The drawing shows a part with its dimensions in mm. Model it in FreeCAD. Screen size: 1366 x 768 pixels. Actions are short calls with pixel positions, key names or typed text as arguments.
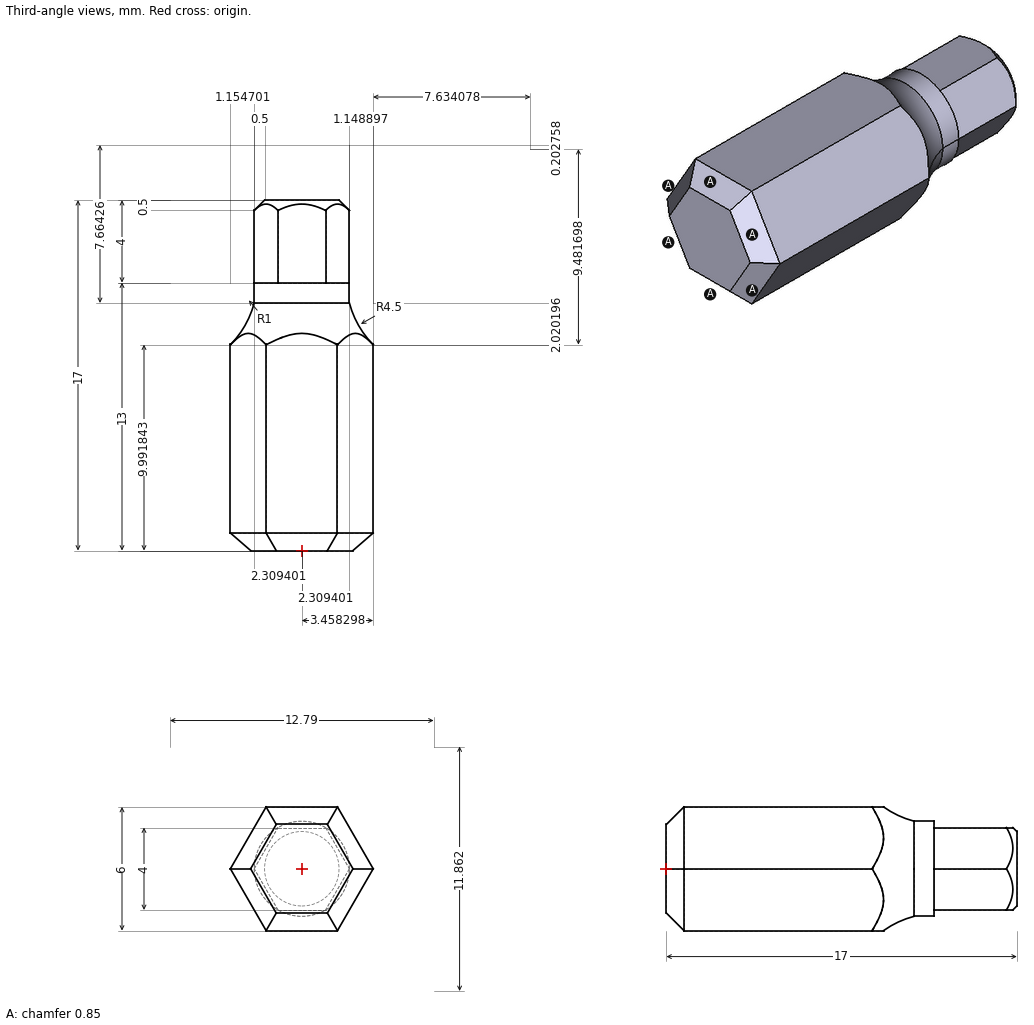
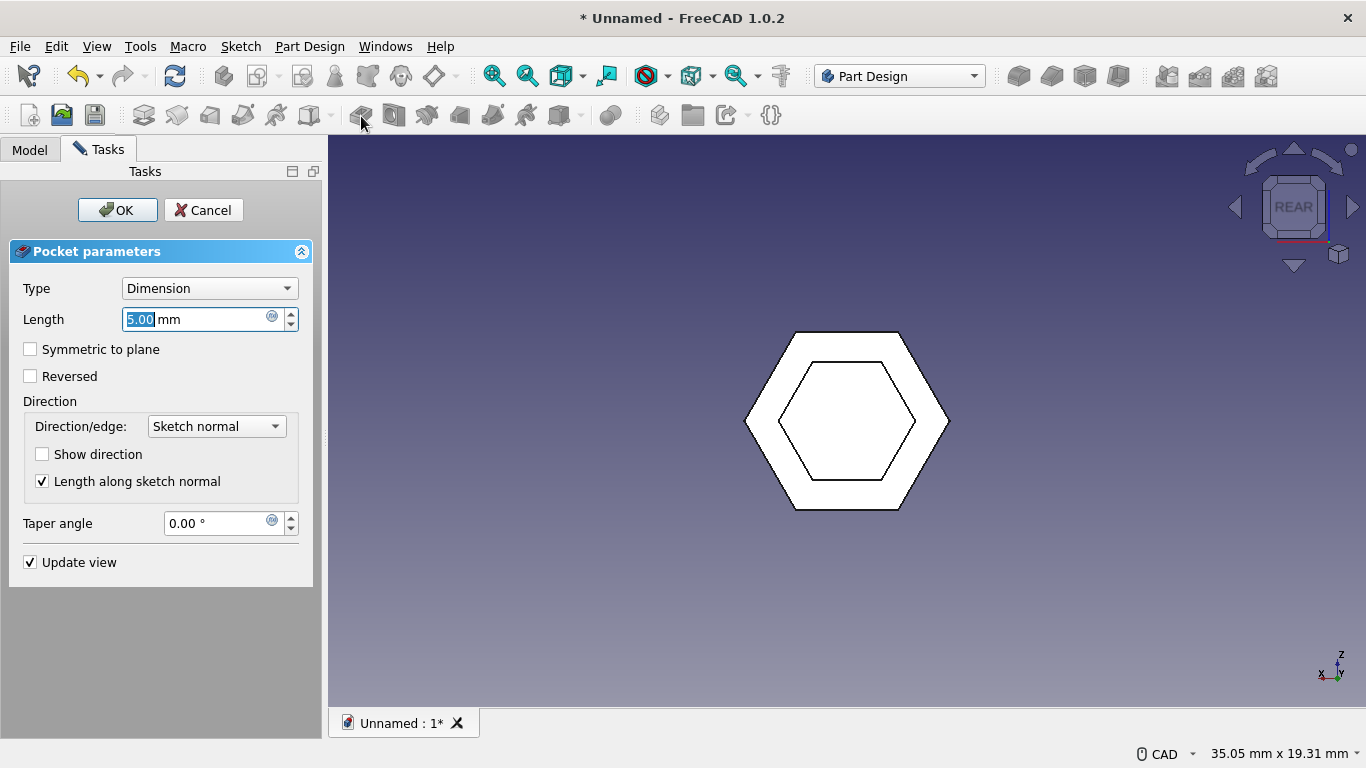
text(4)
key(Tab)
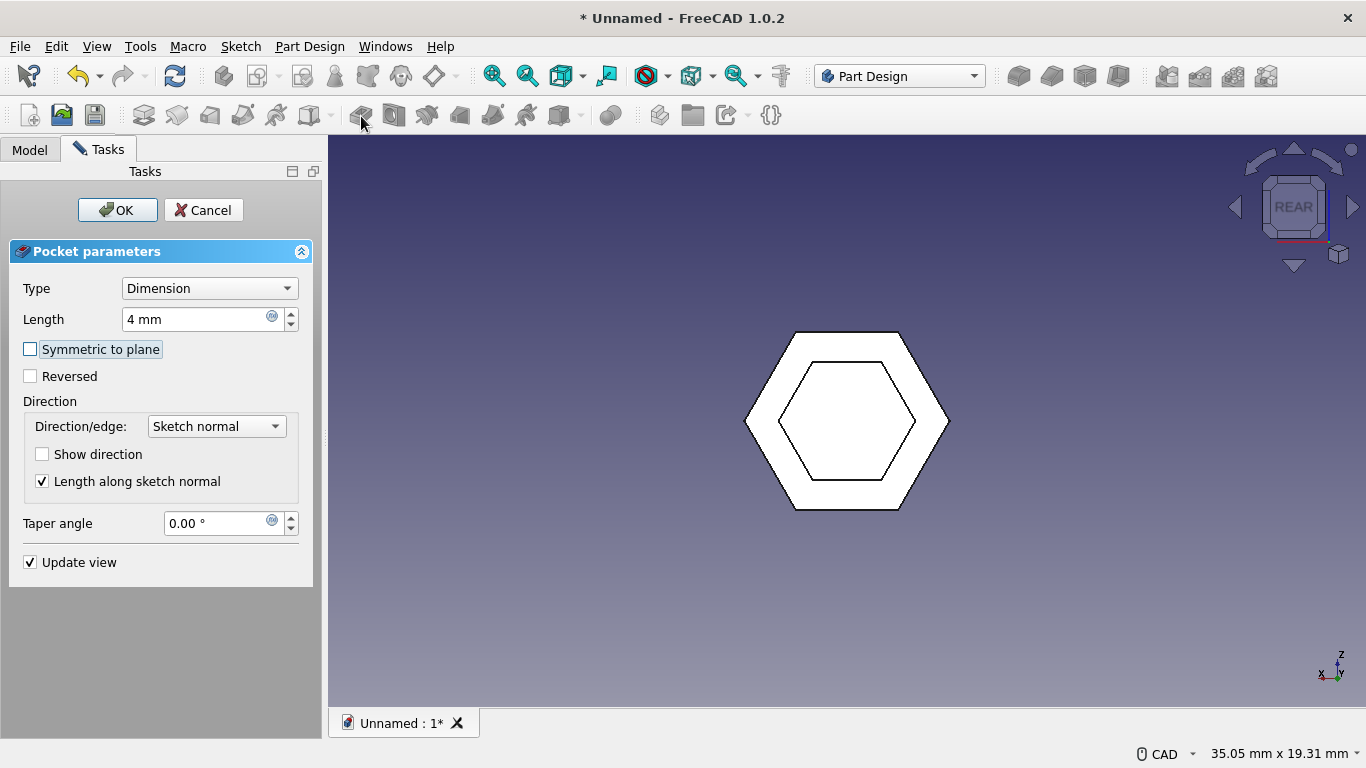
click(118, 210)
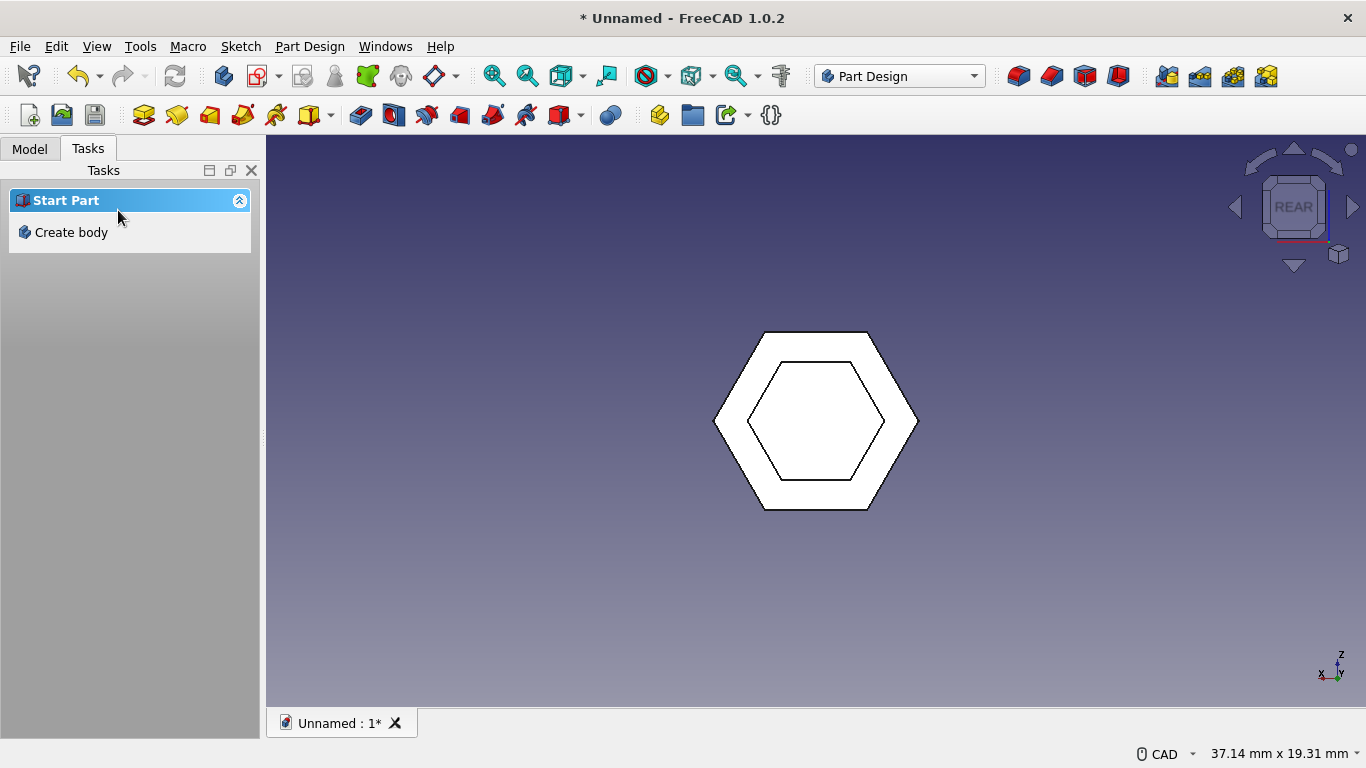
click(495, 76)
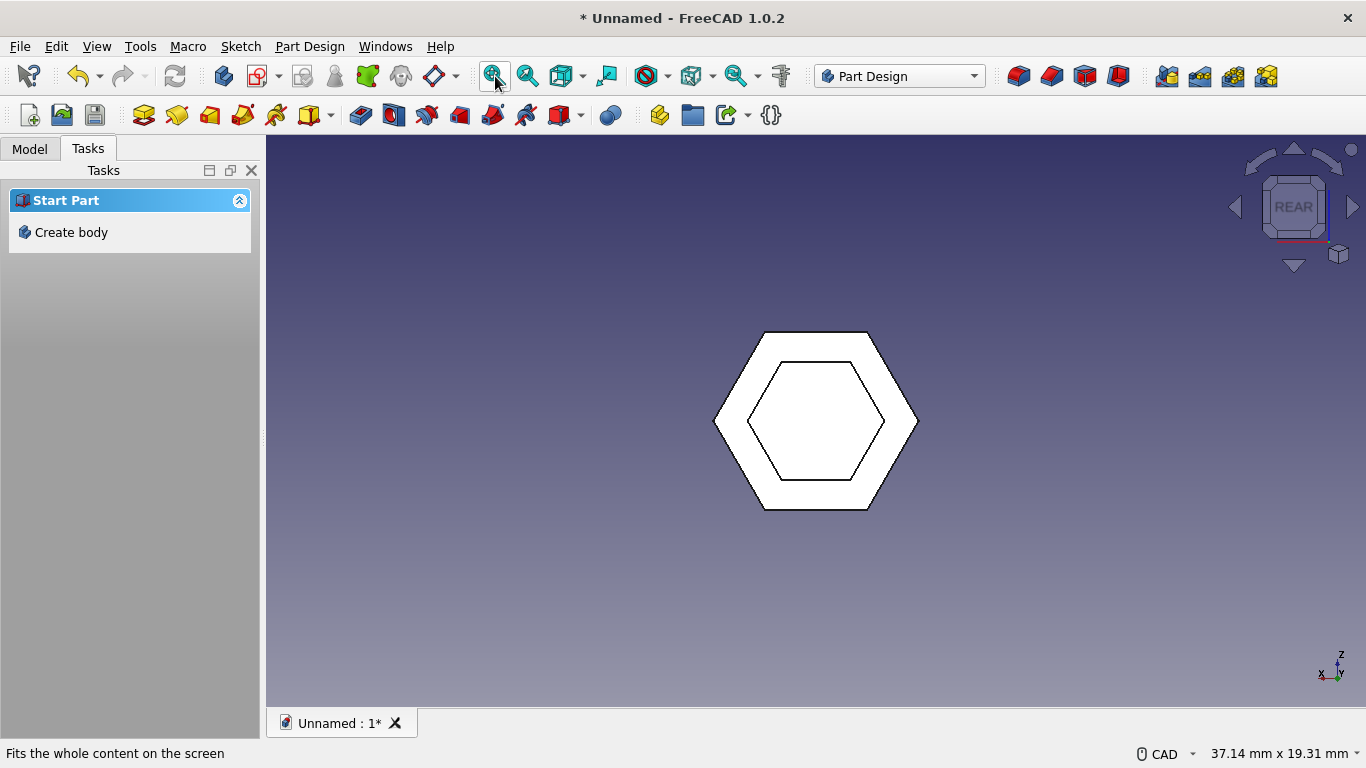
click(256, 76)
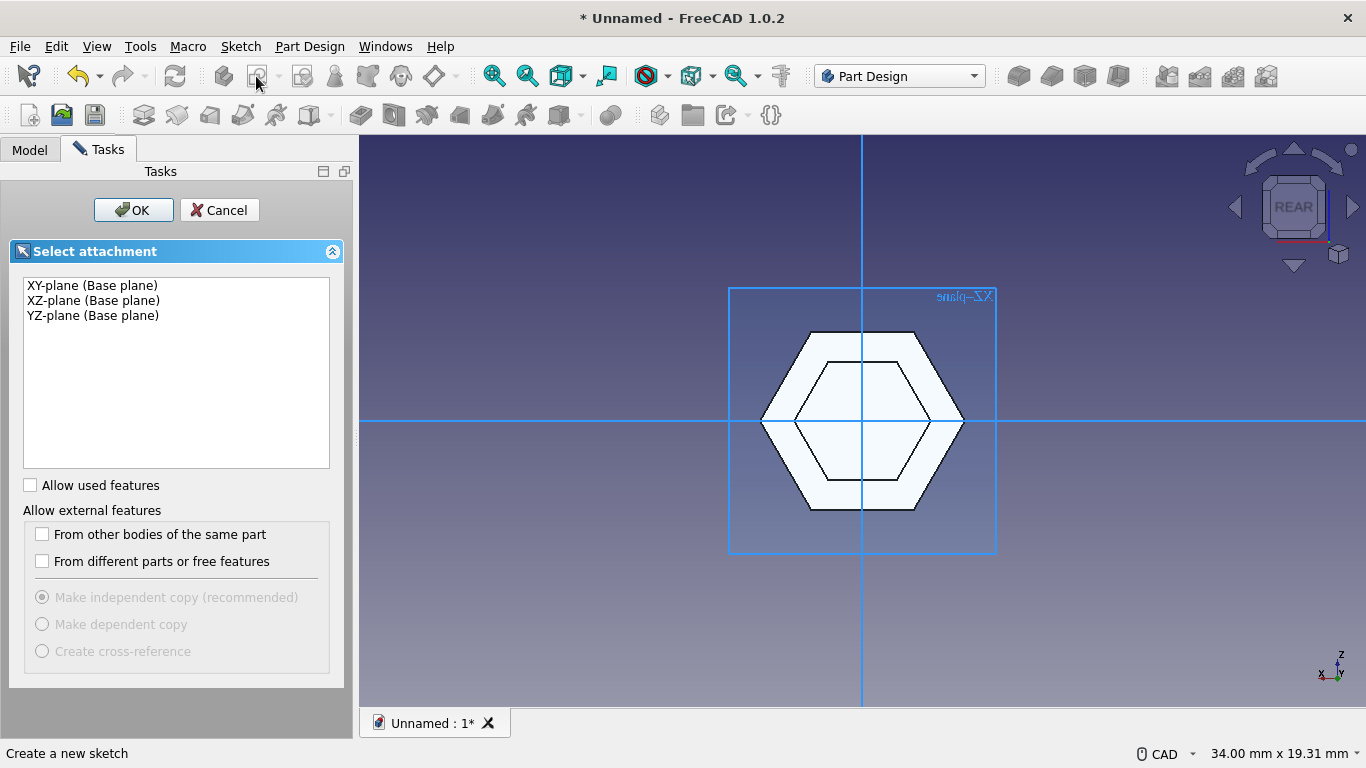
click(84, 286)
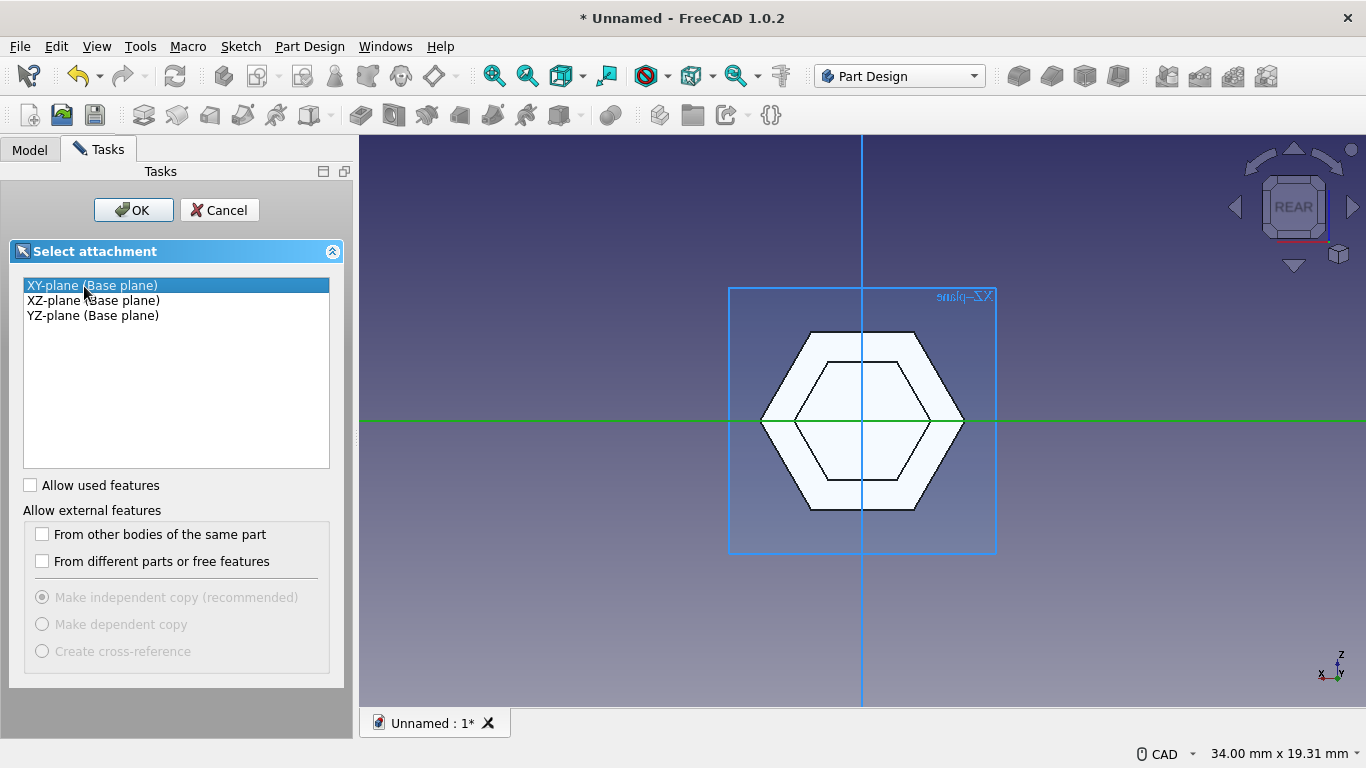
click(134, 210)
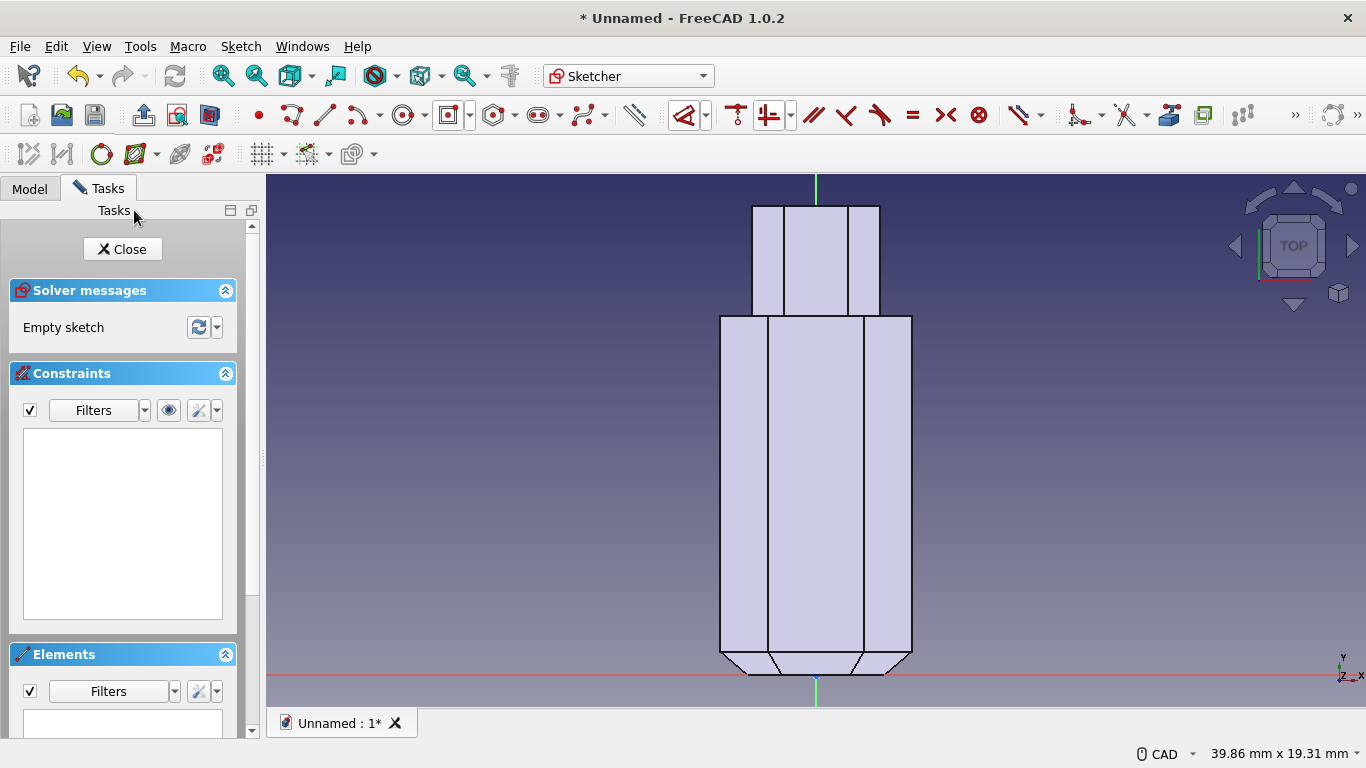
click(210, 116)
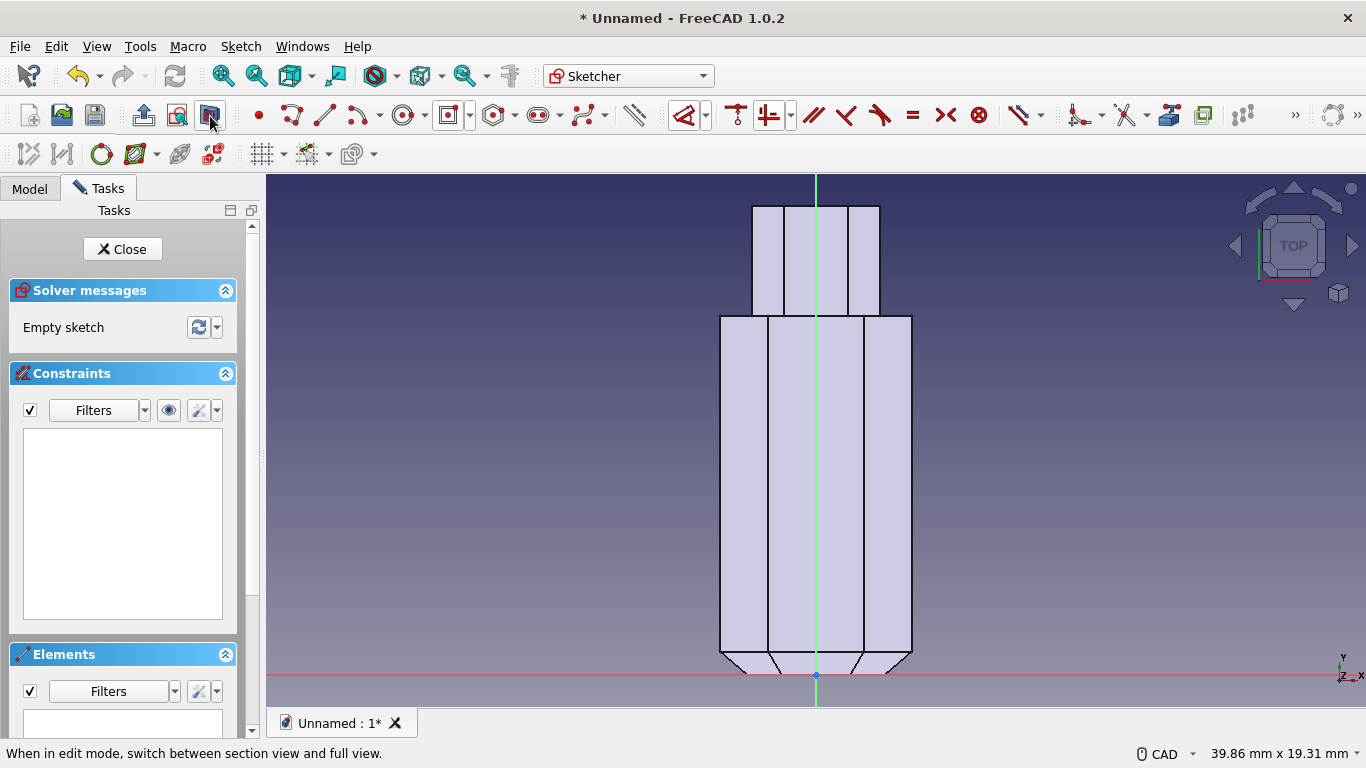
scroll(438, 202, down, 1)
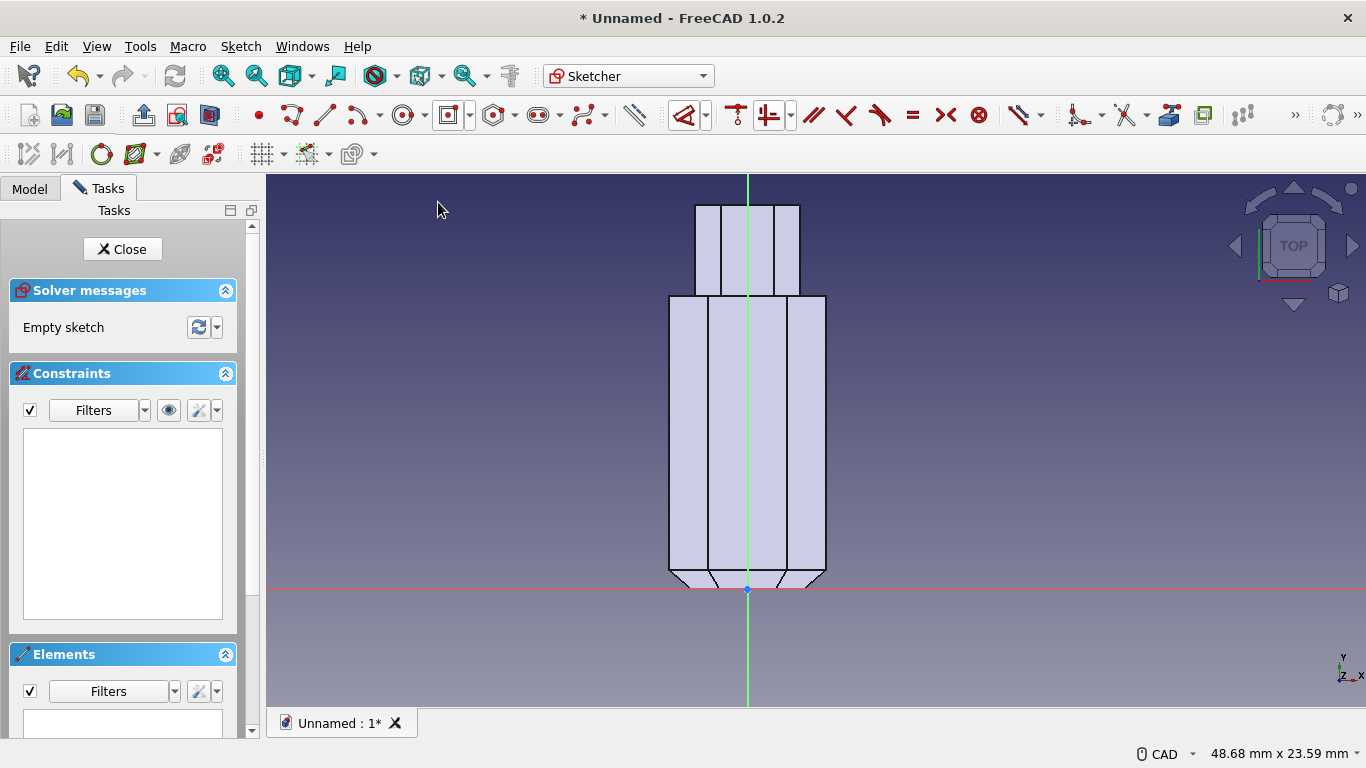
click(292, 116)